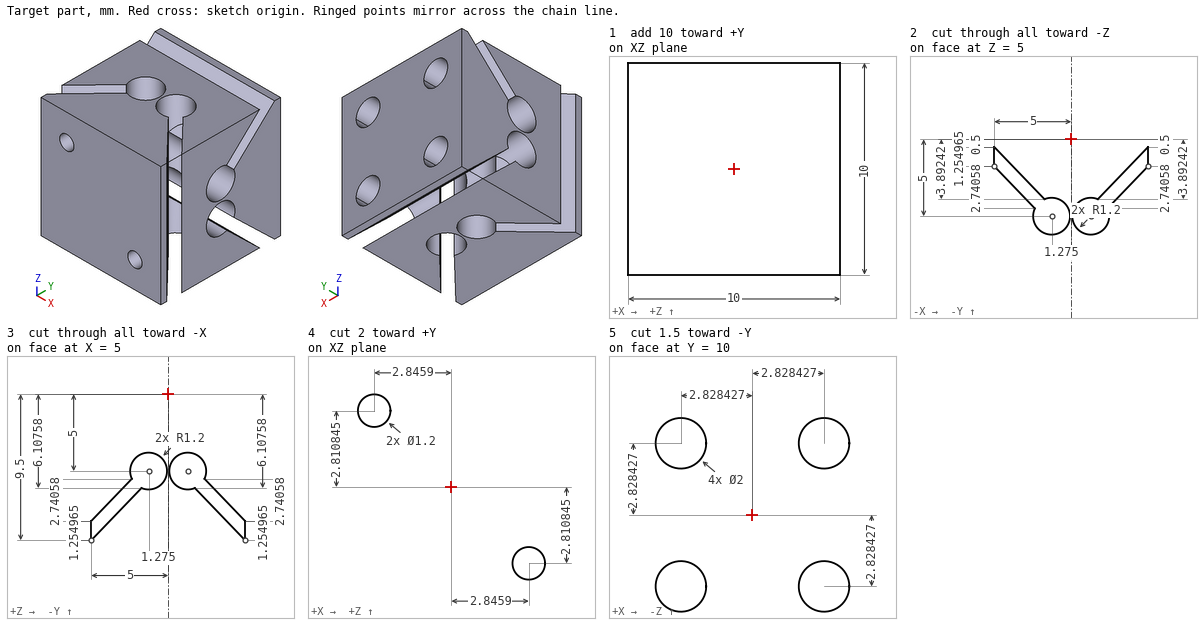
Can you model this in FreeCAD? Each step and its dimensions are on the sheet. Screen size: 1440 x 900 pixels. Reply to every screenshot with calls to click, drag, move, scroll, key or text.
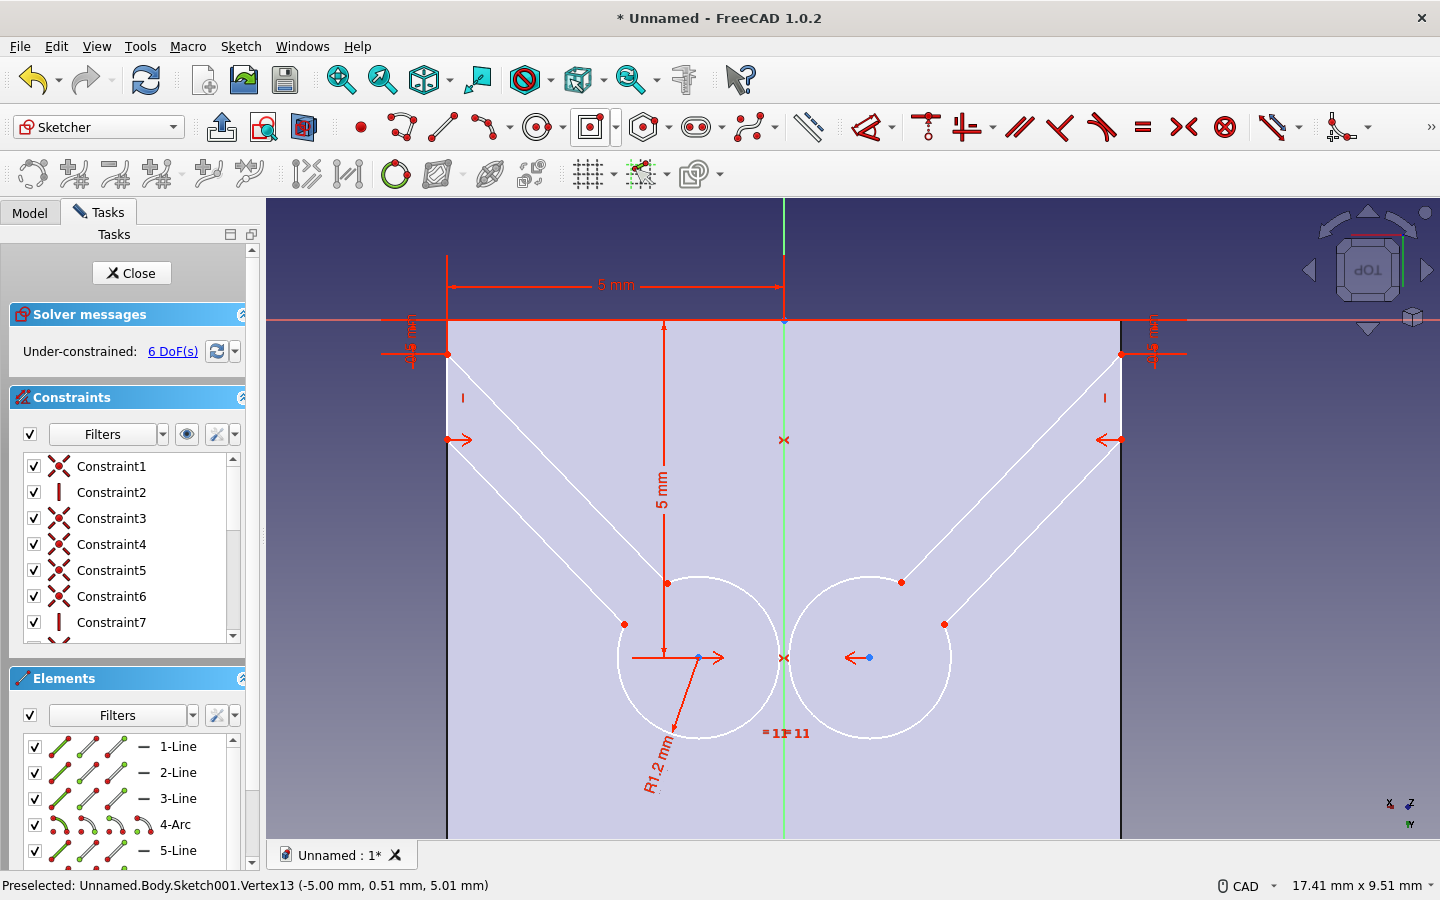
click(699, 658)
click(741, 286)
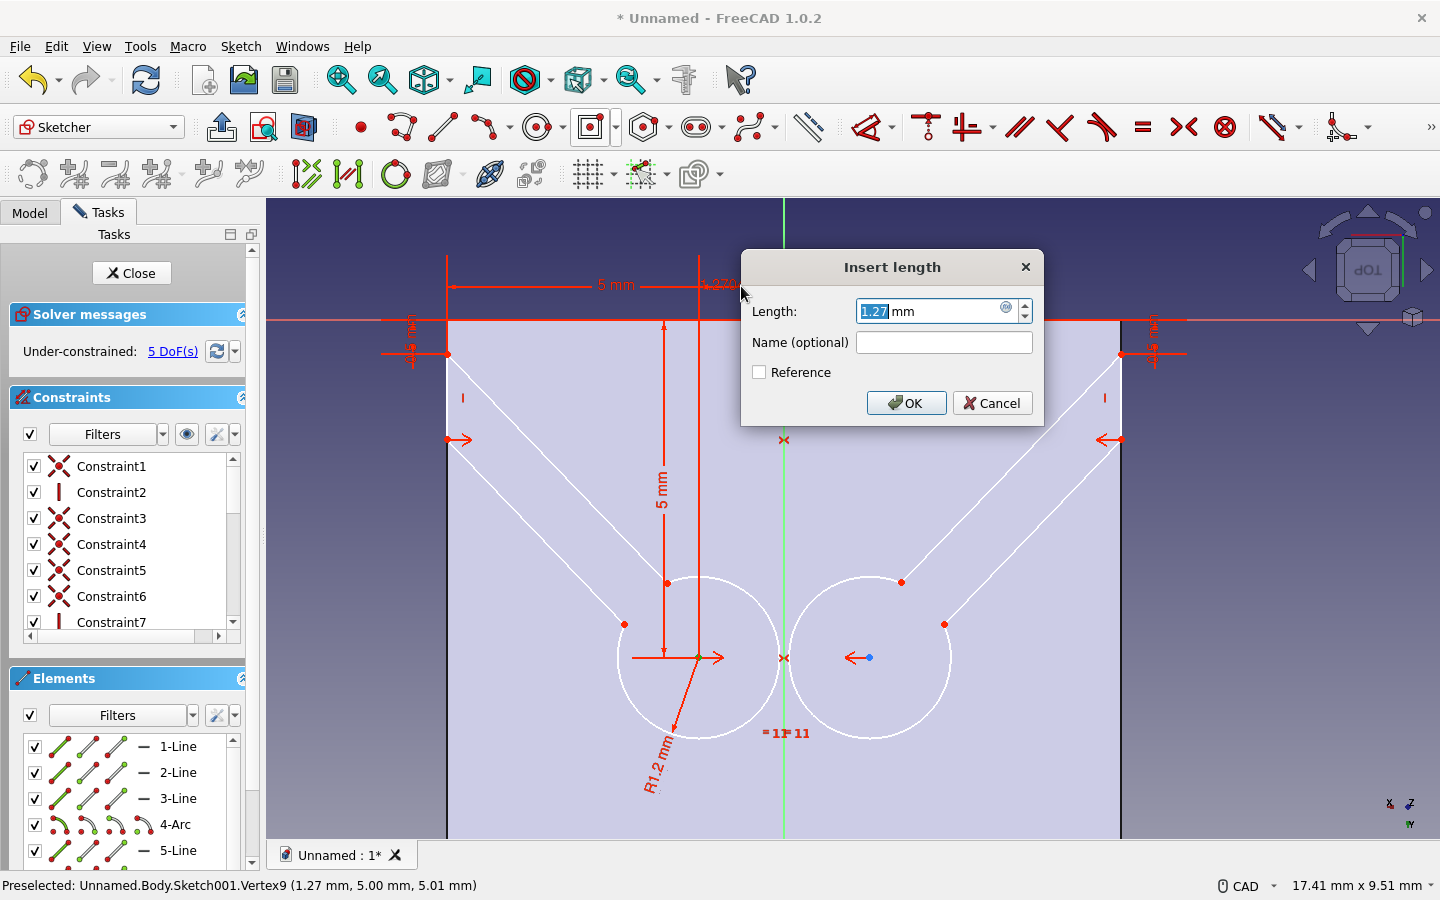
text(1.275)
key(Return)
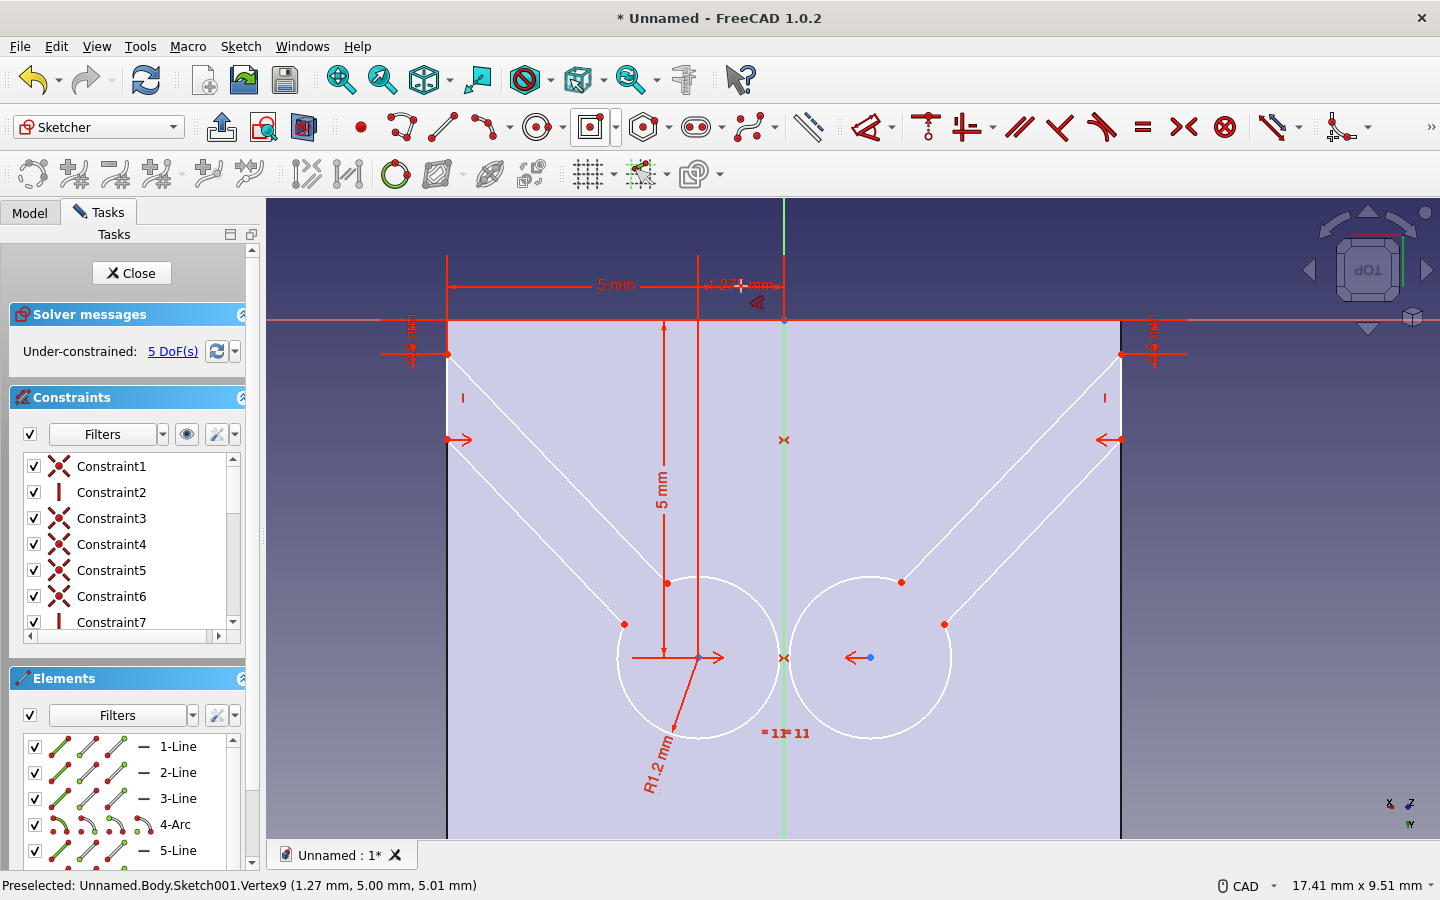
click(447, 380)
click(413, 397)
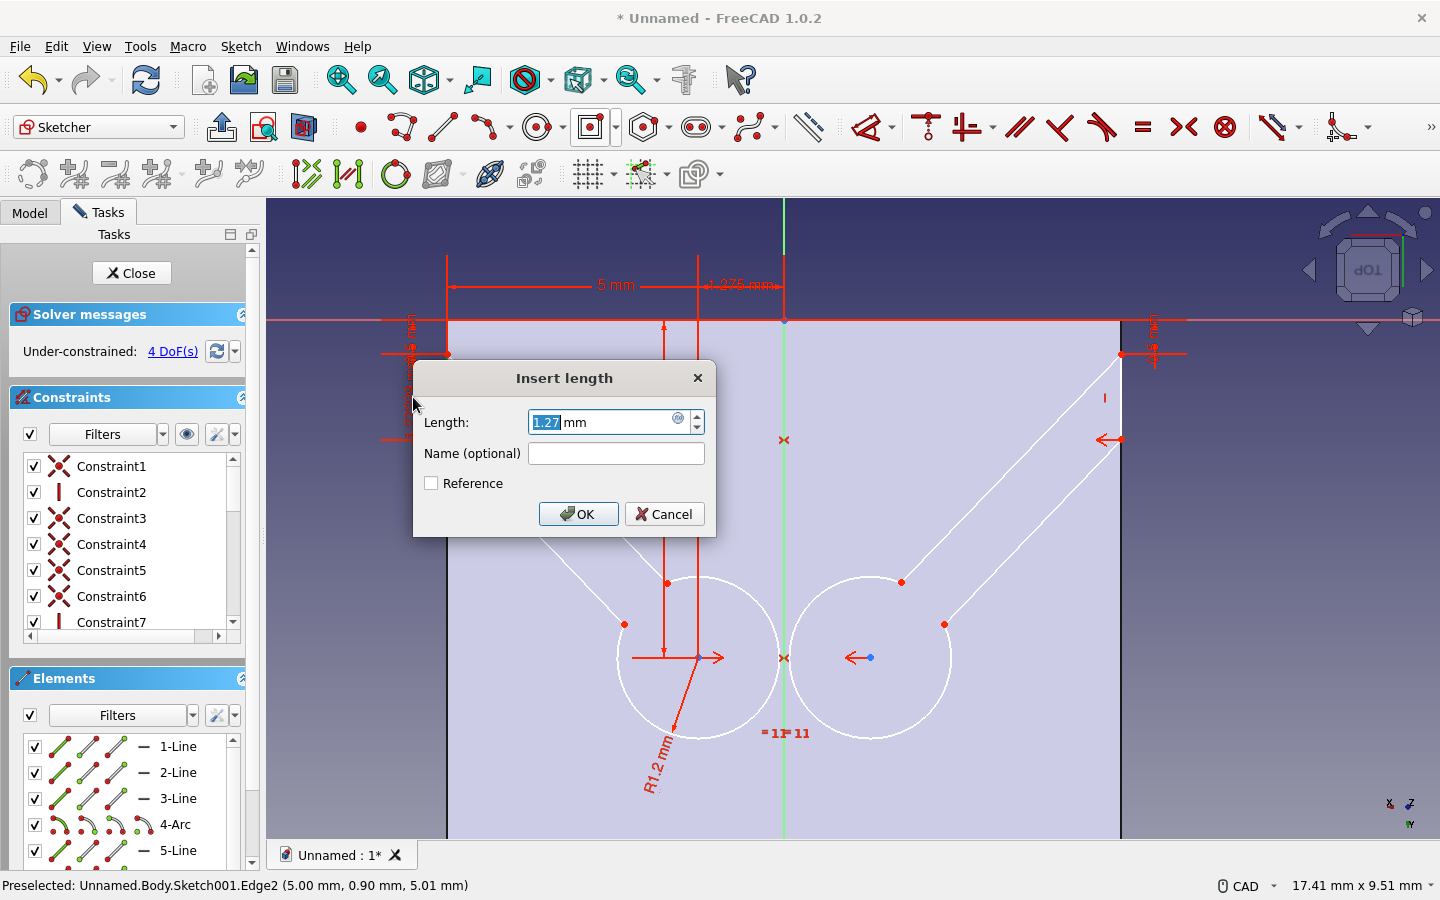
text(1.254965)
key(Return)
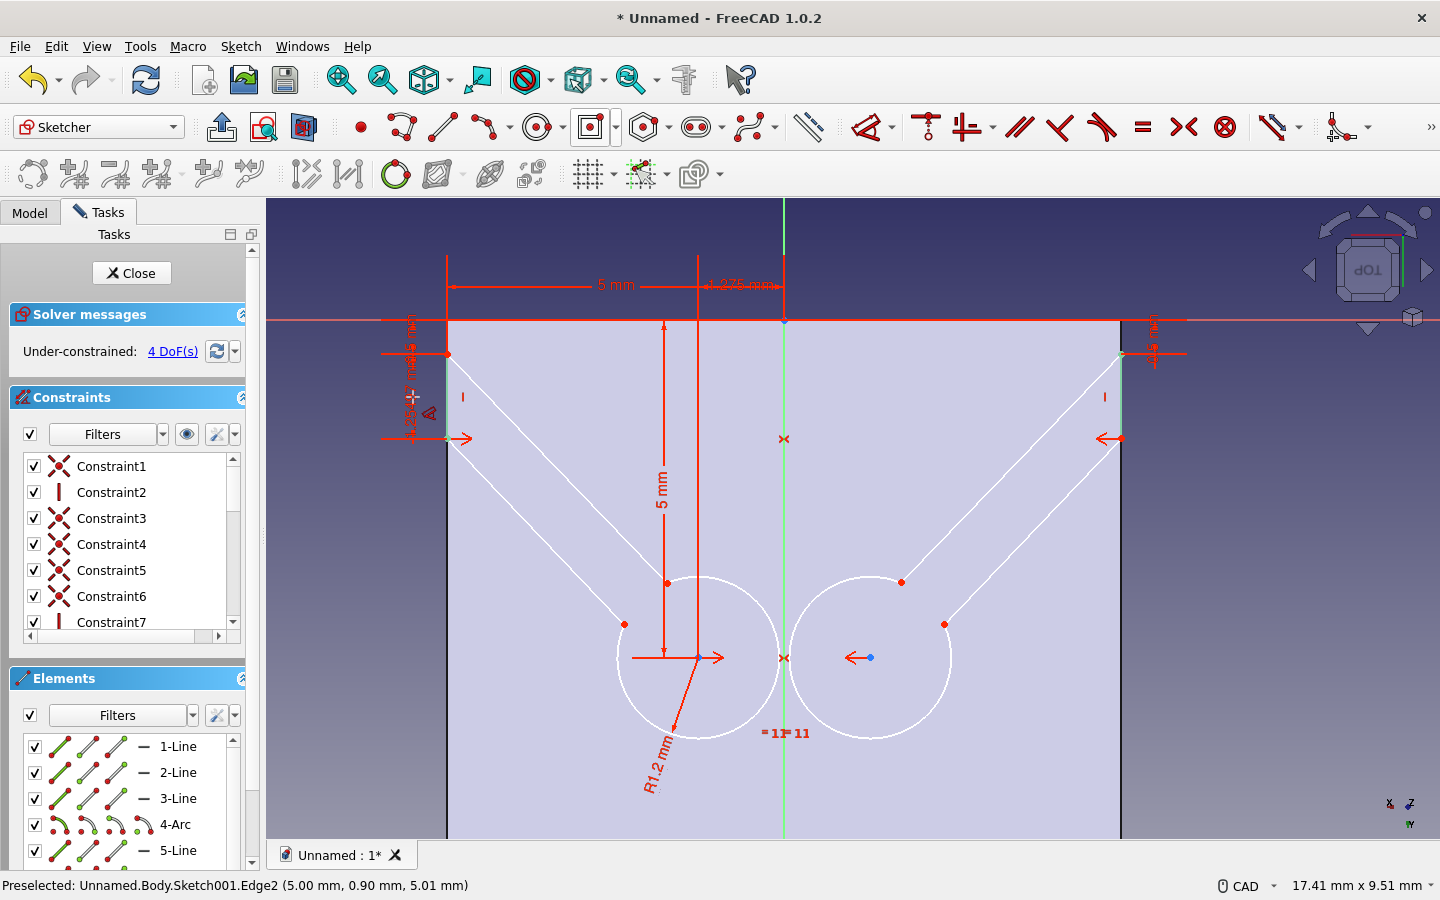
click(667, 583)
click(633, 452)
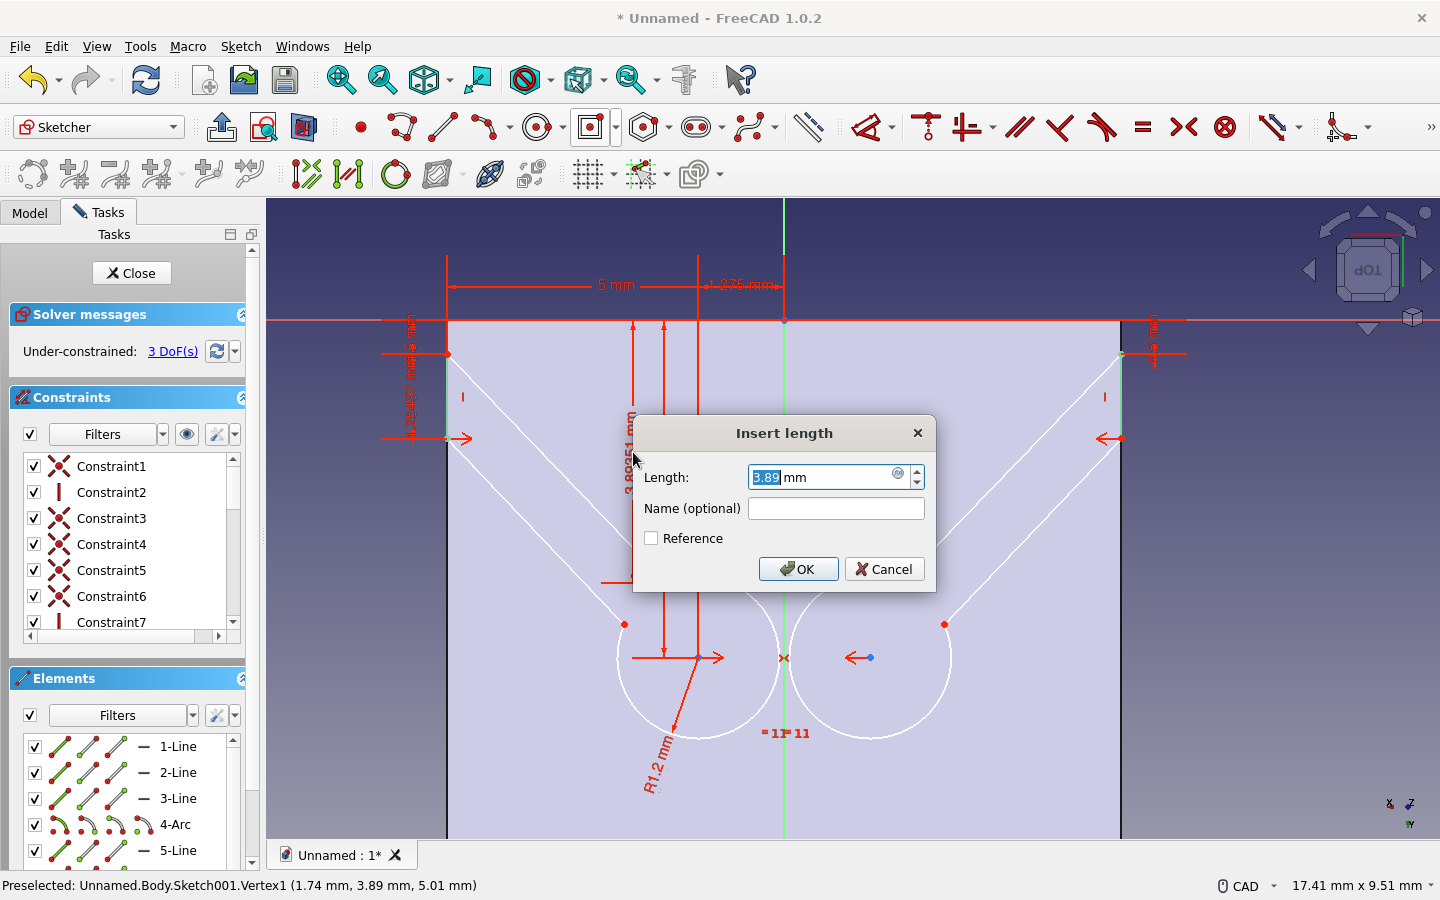
text(3.89242)
key(Return)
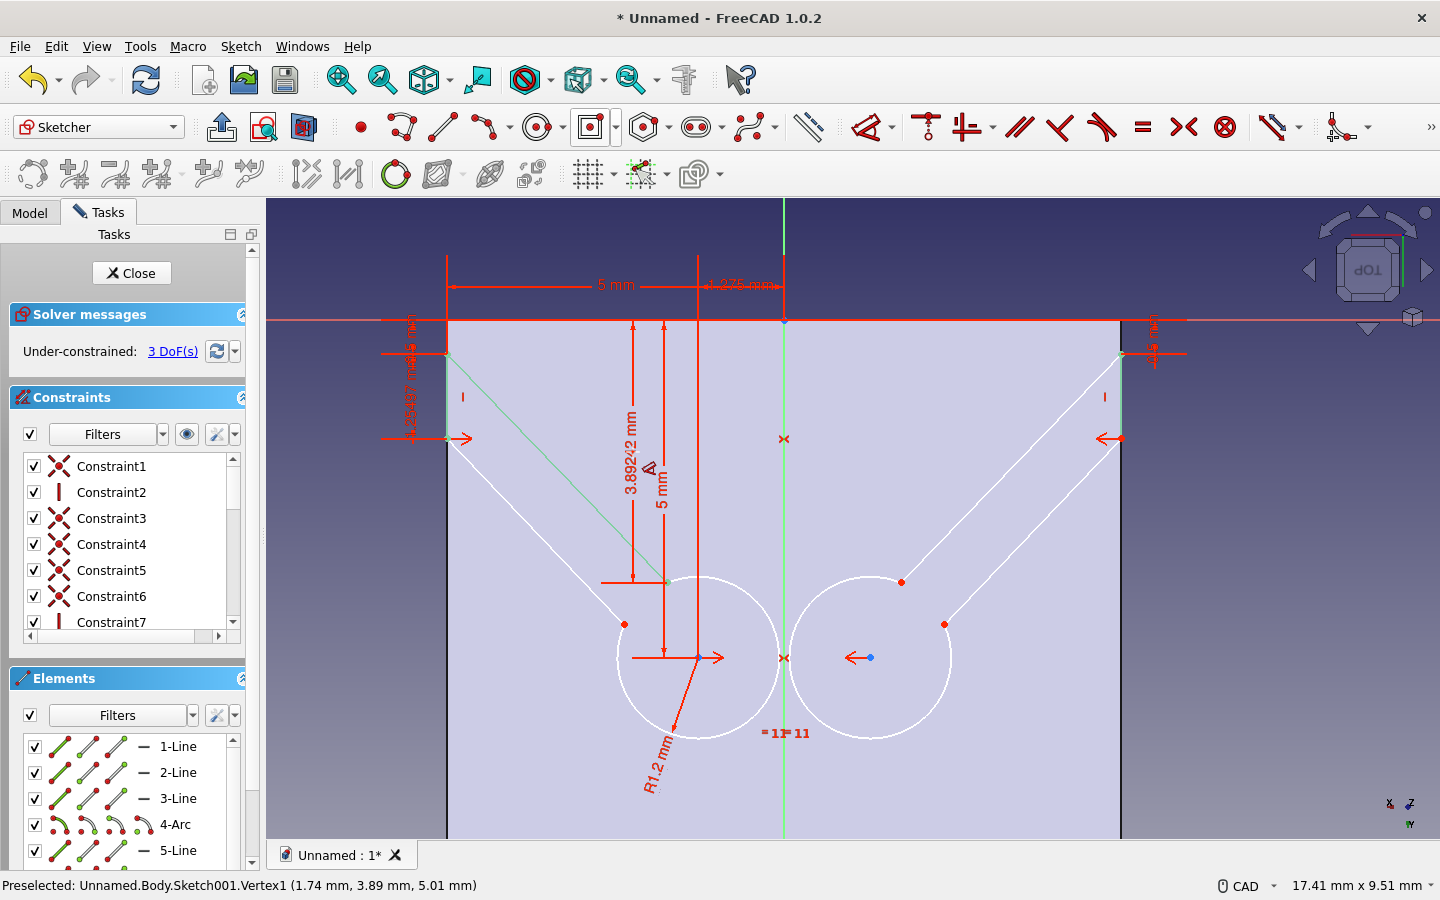
click(901, 583)
click(935, 452)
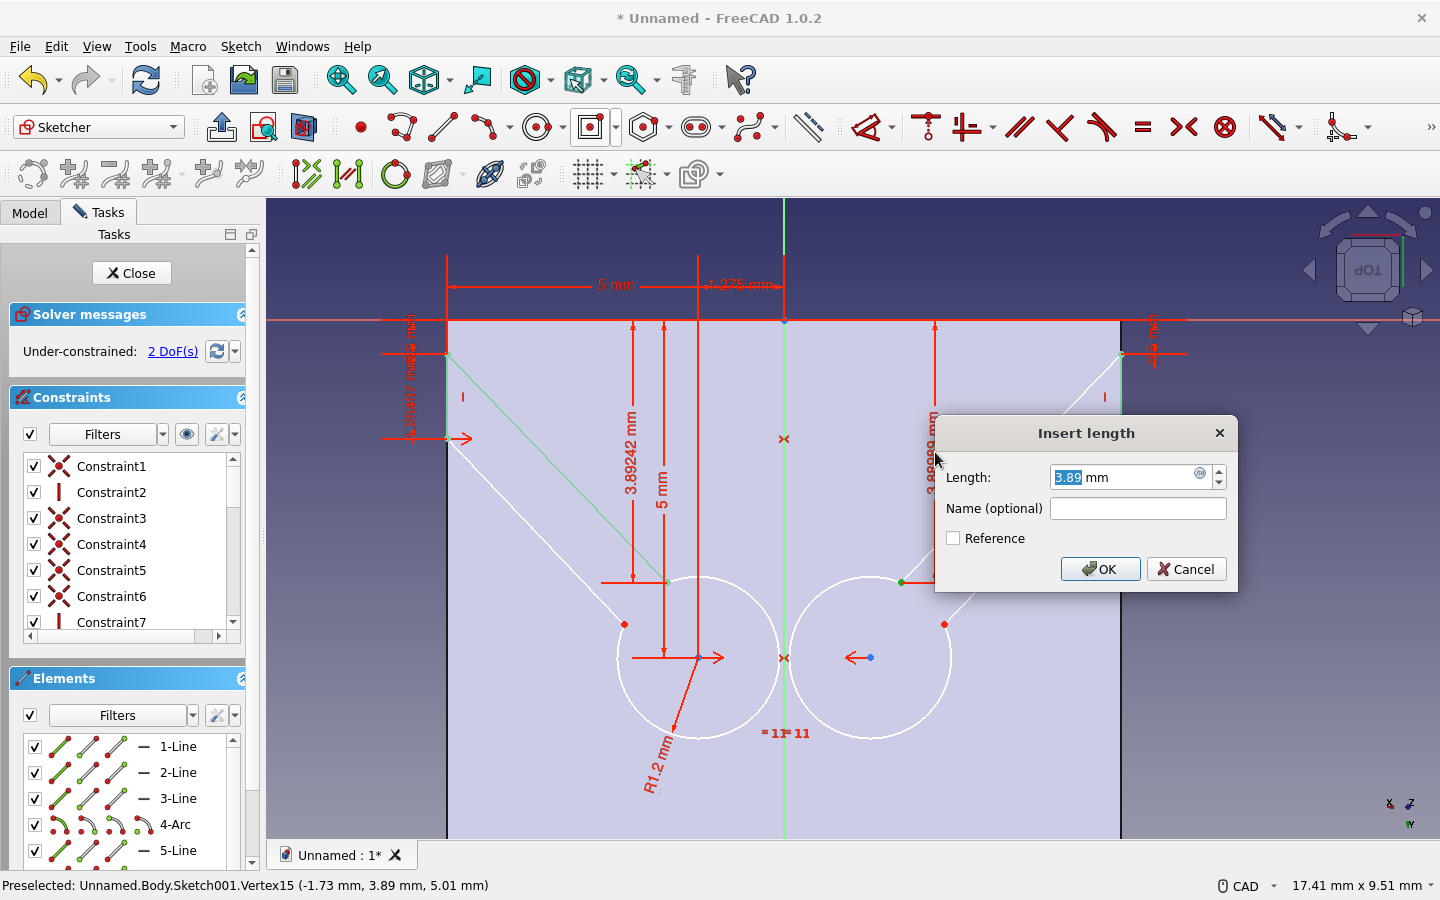
text(3.89242)
key(Return)